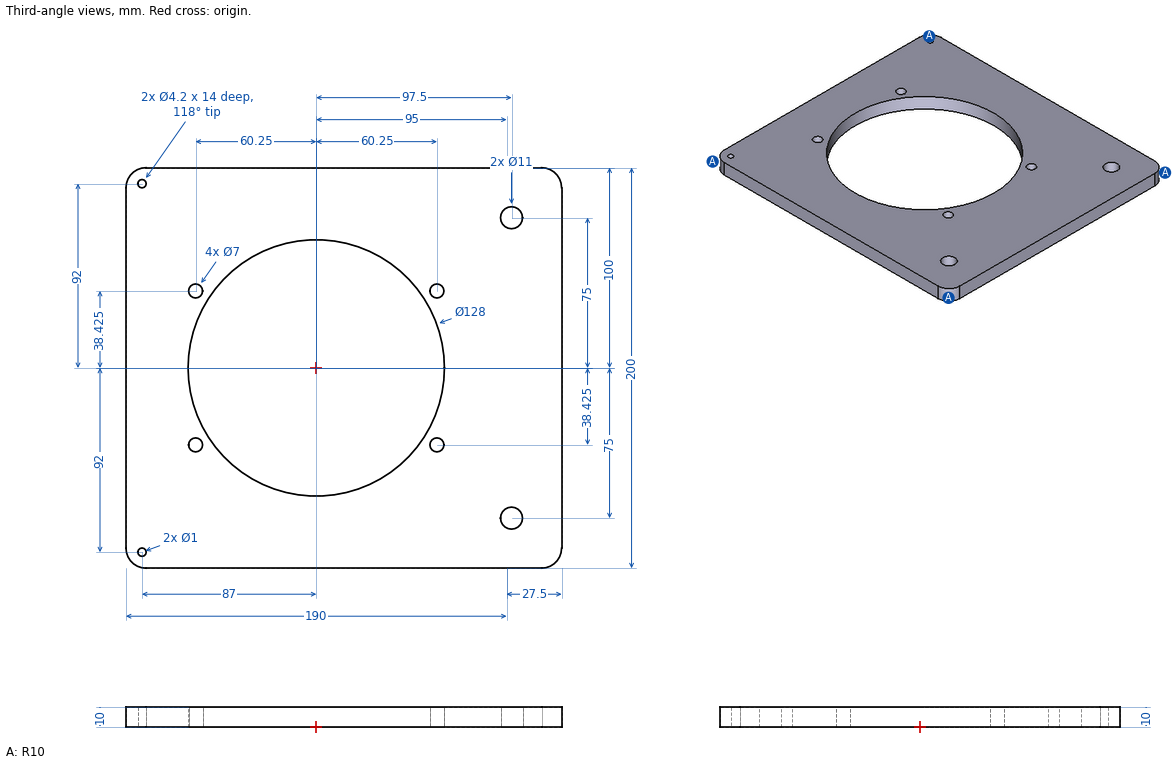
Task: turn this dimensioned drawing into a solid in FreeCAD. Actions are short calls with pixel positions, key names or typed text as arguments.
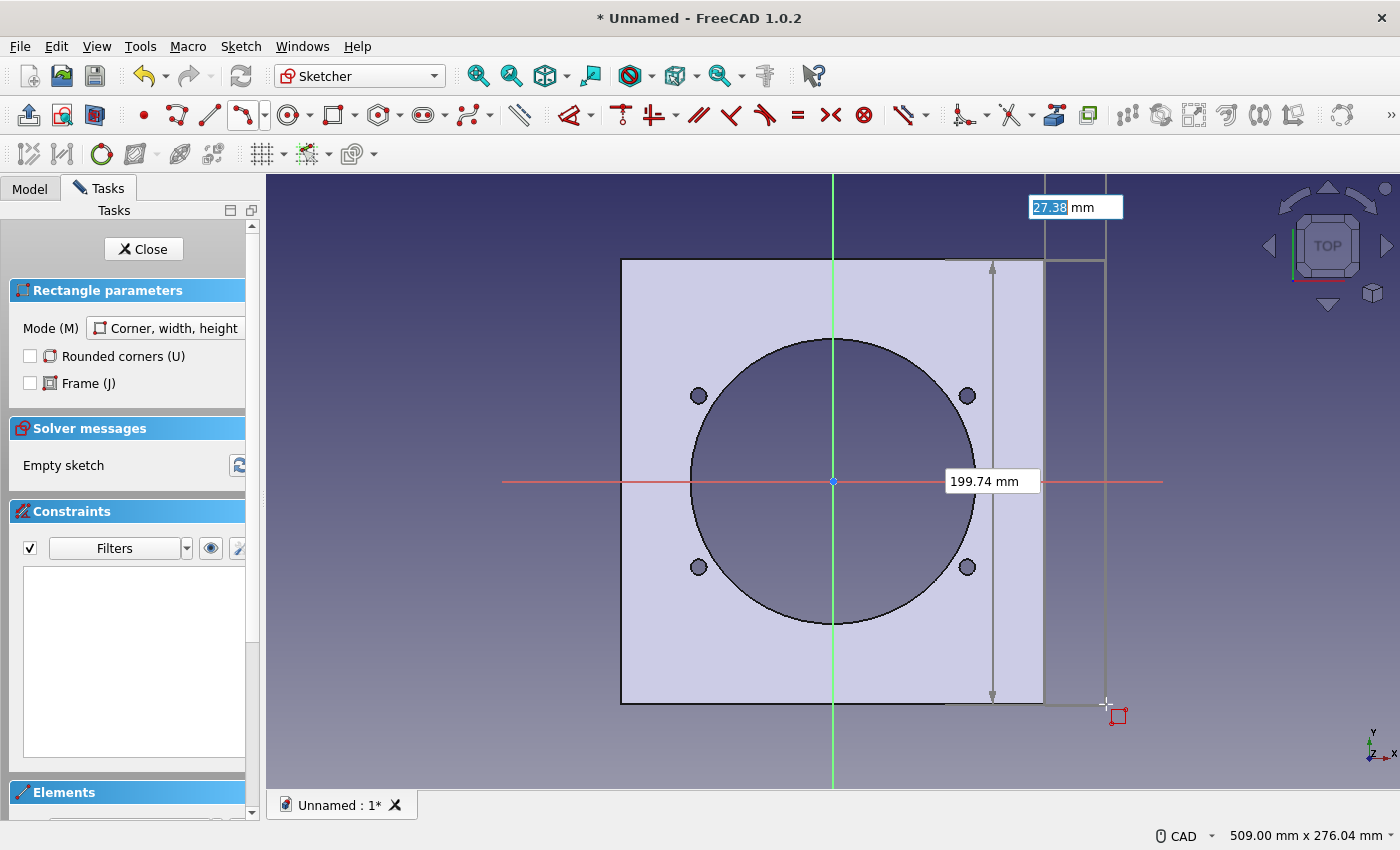
text(27.5)
key(Tab)
text(200)
key(Return)
key(Escape)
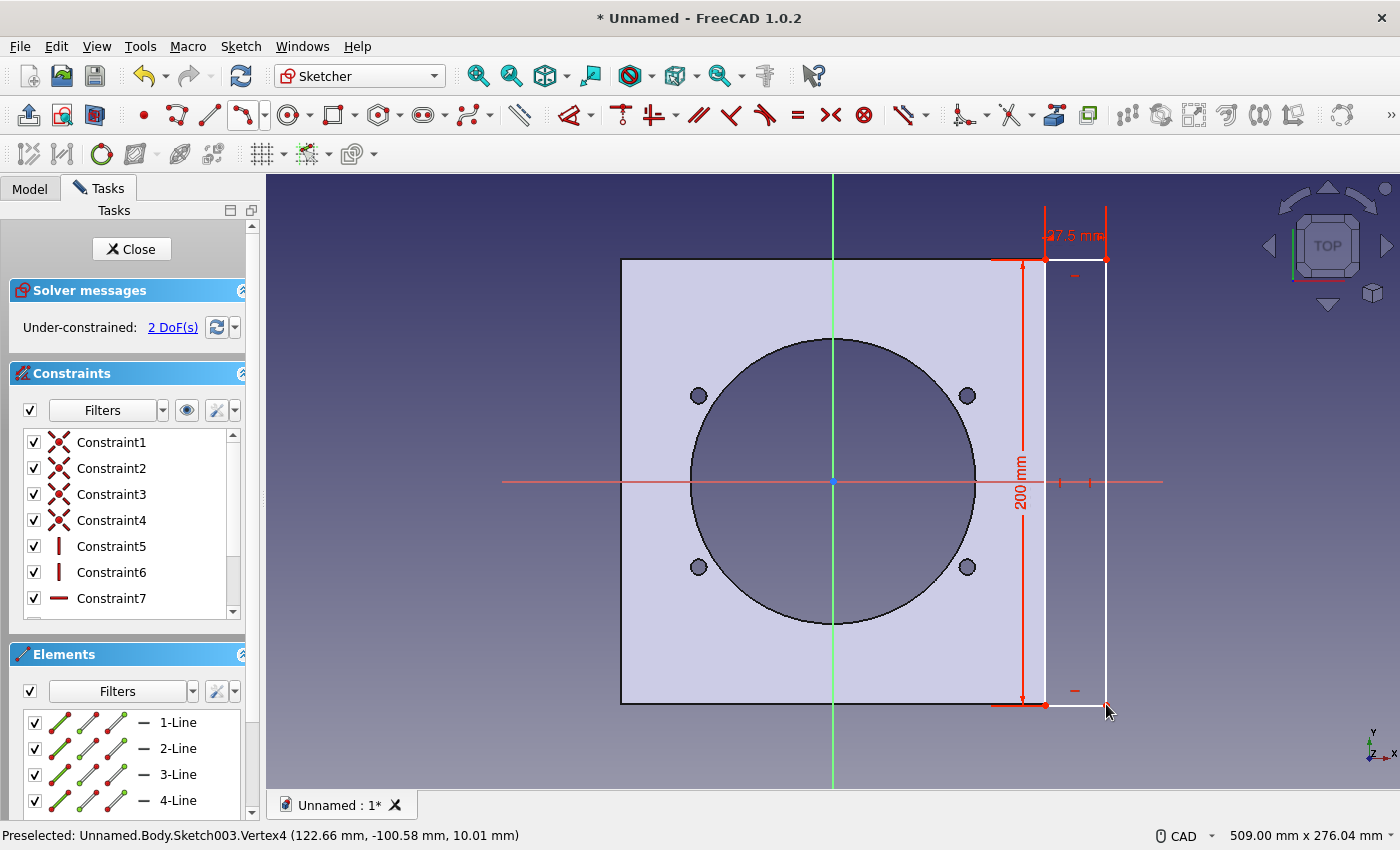
key(d)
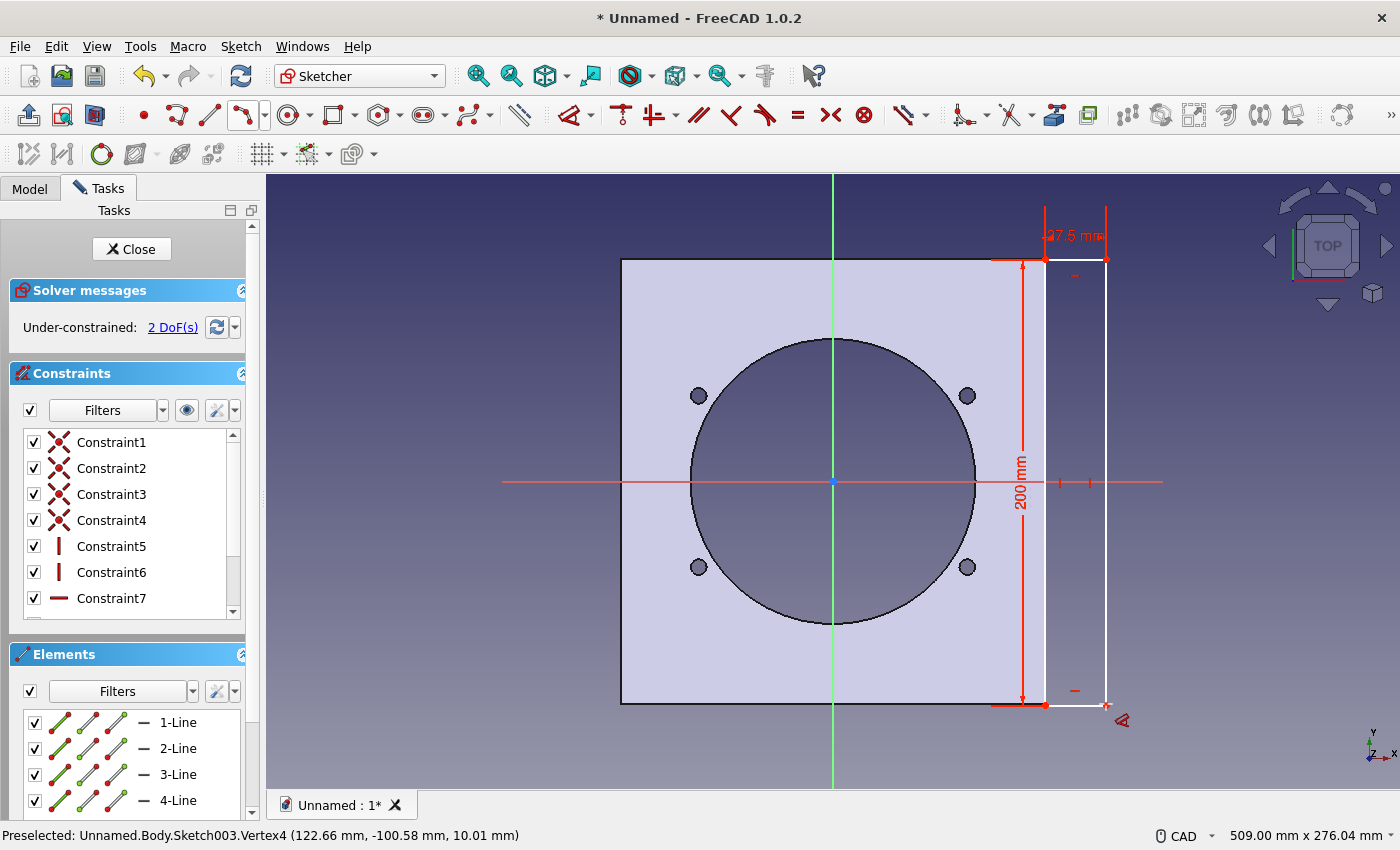
click(1045, 260)
click(939, 226)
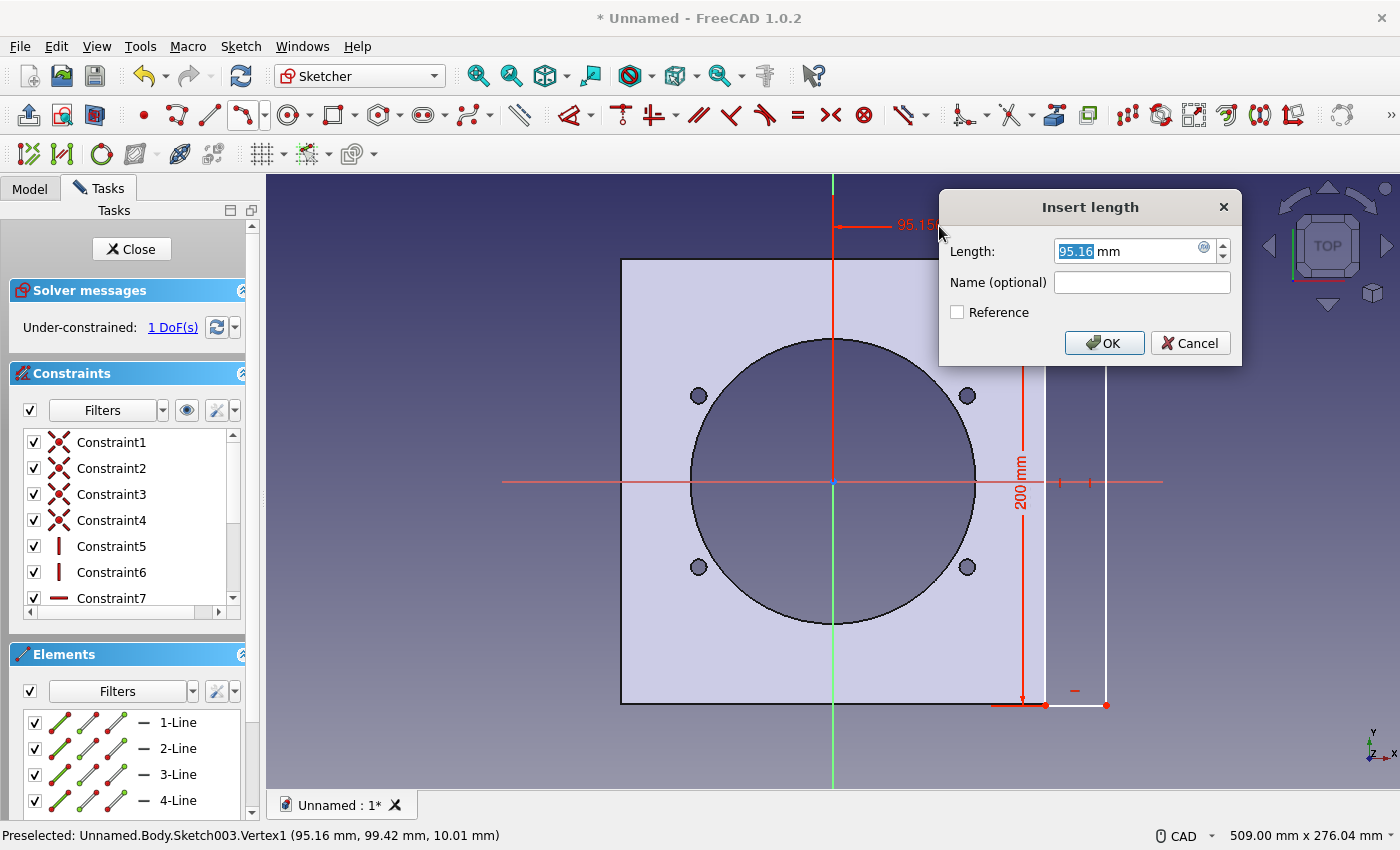
text(95)
key(Return)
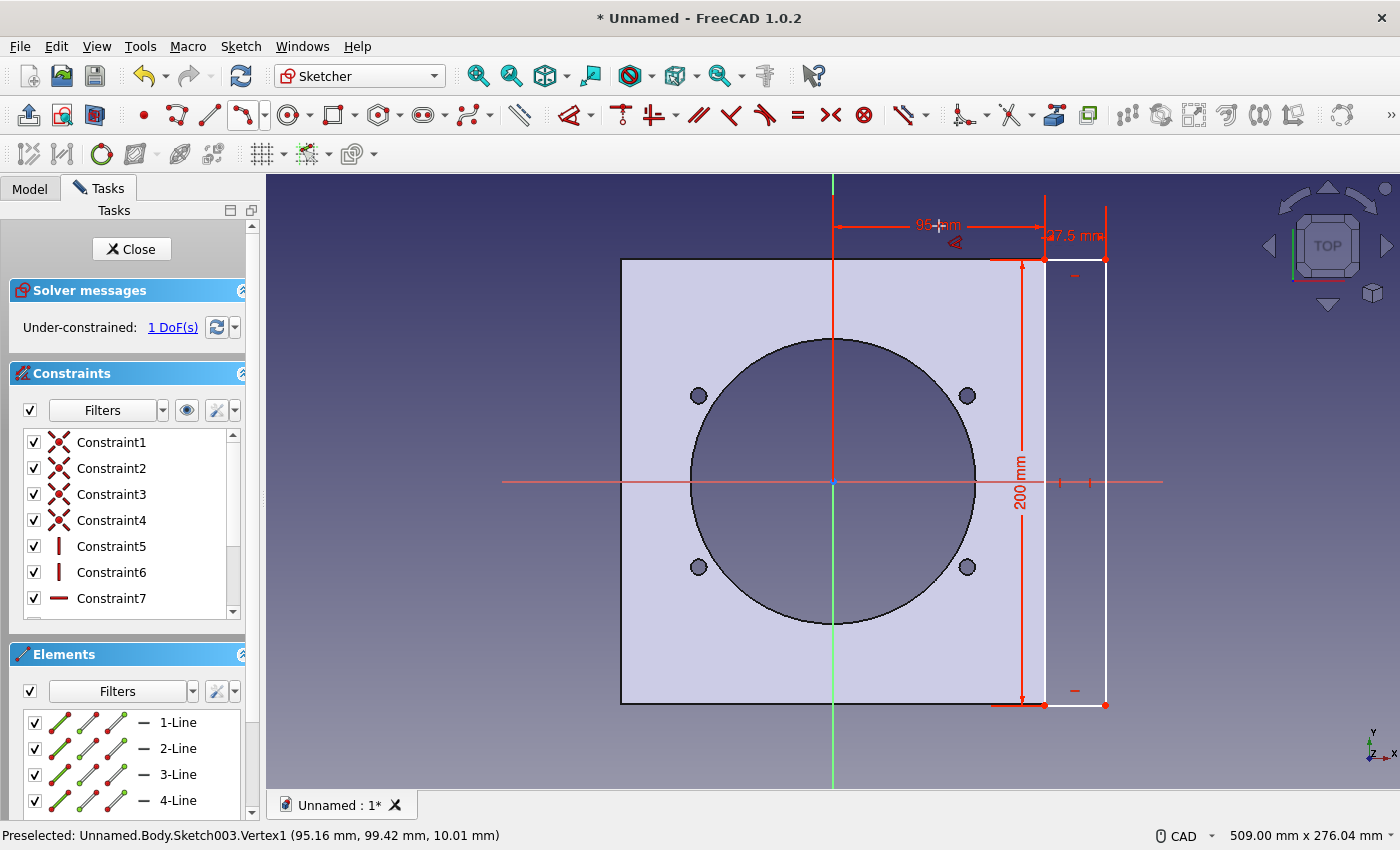
click(1045, 260)
click(799, 371)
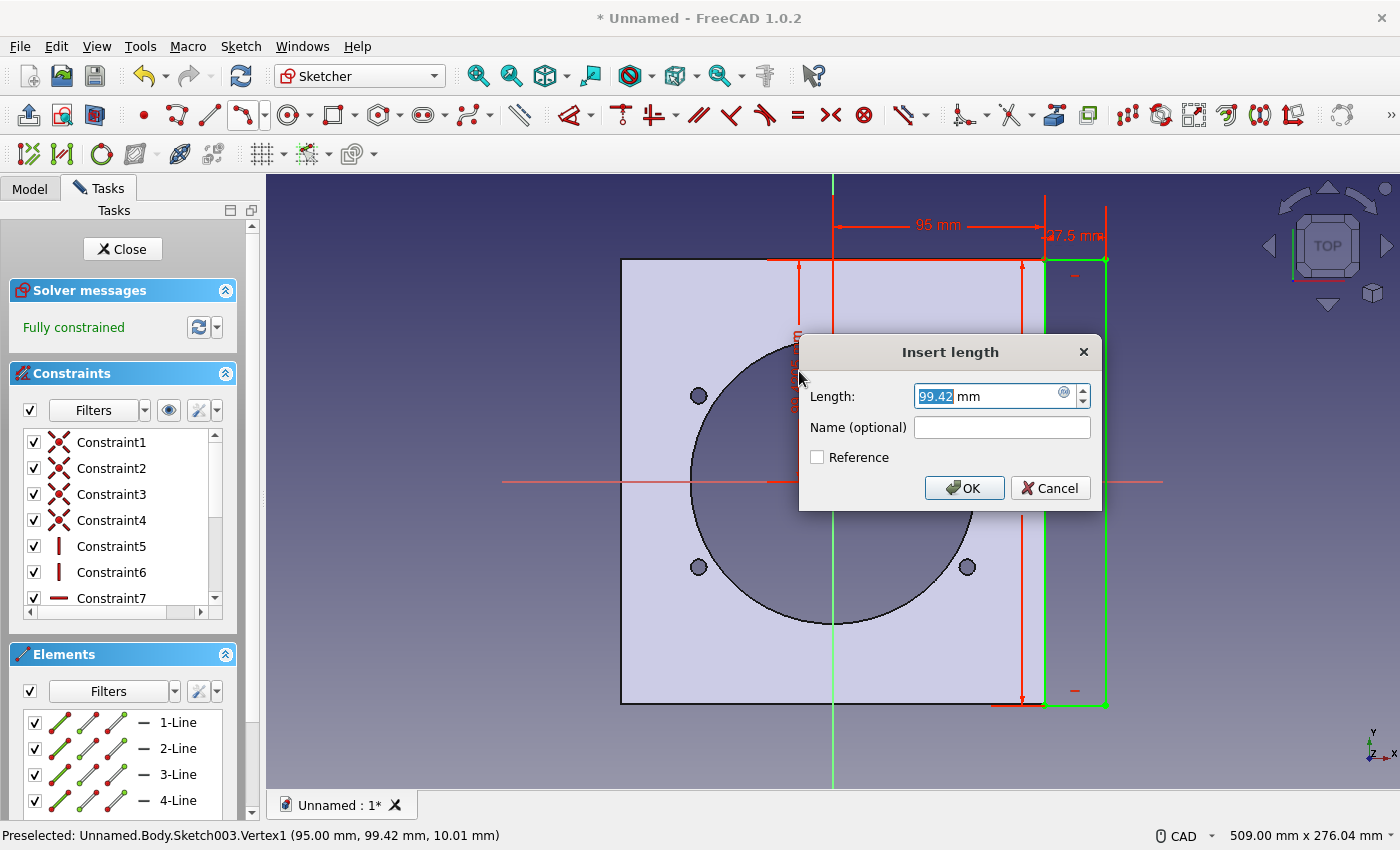
text(100)
key(Return)
key(Escape)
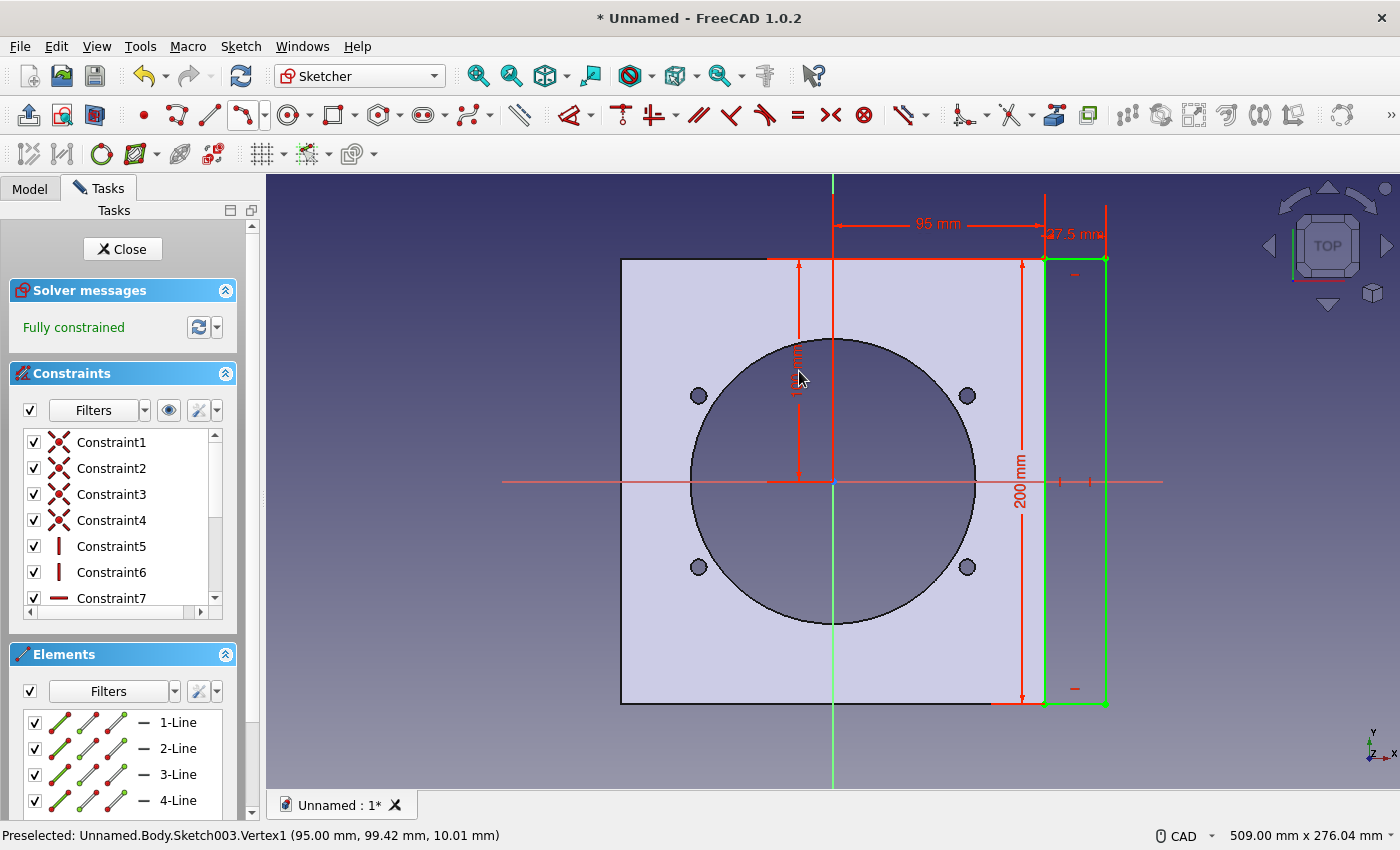
click(123, 249)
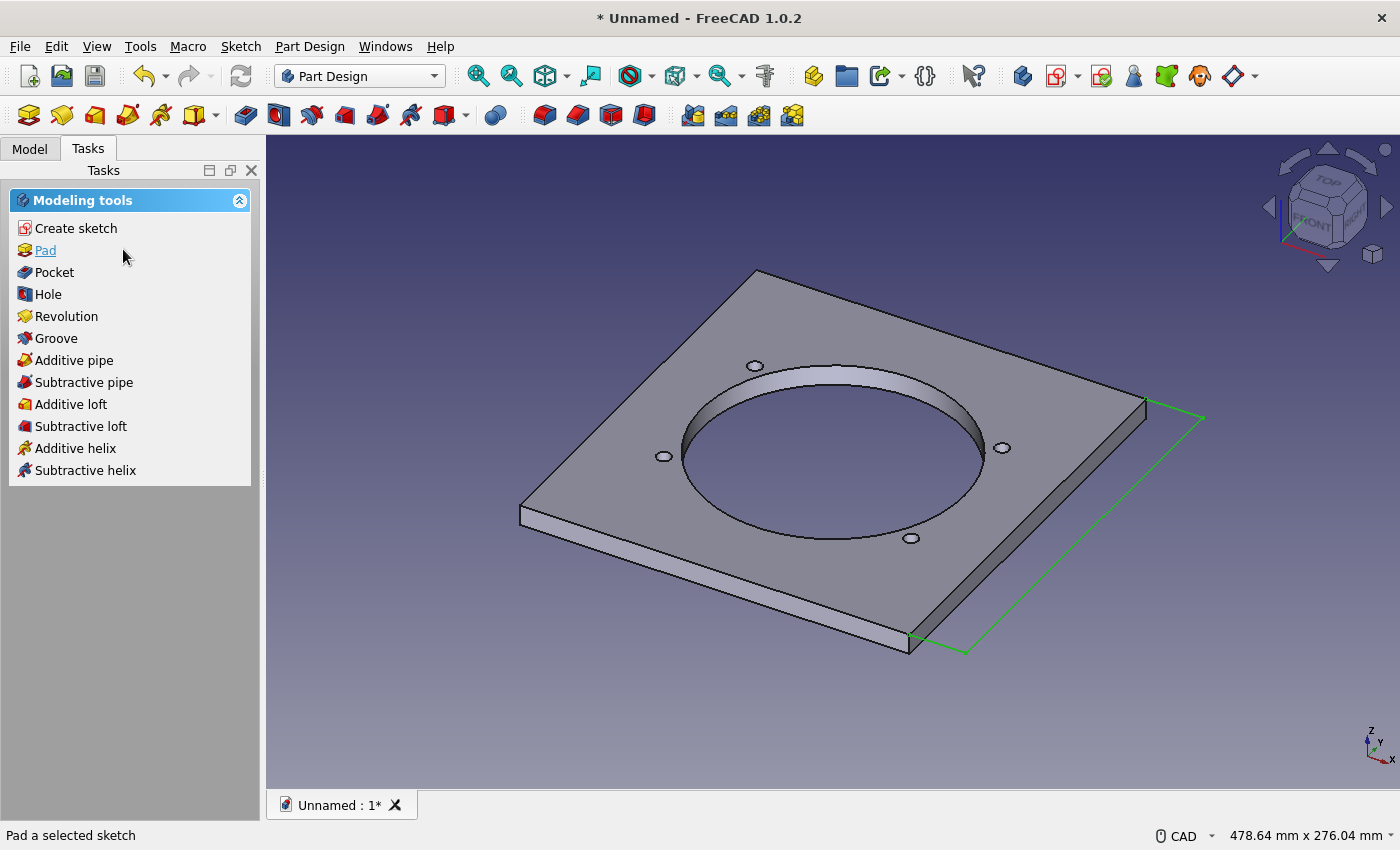
click(29, 116)